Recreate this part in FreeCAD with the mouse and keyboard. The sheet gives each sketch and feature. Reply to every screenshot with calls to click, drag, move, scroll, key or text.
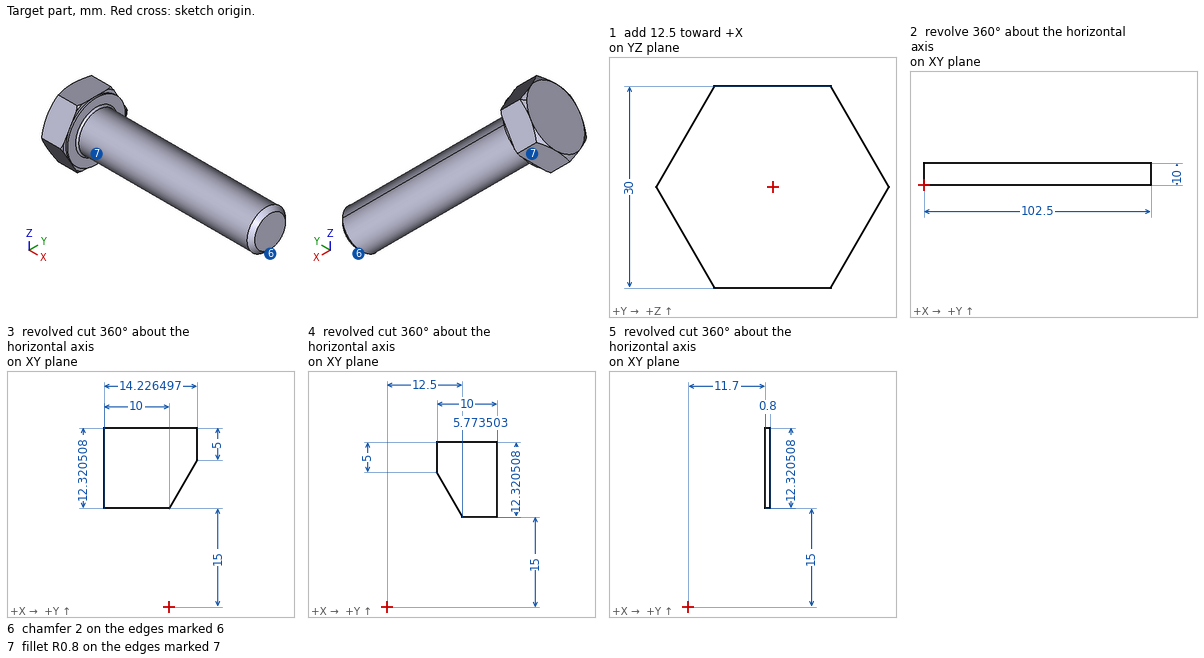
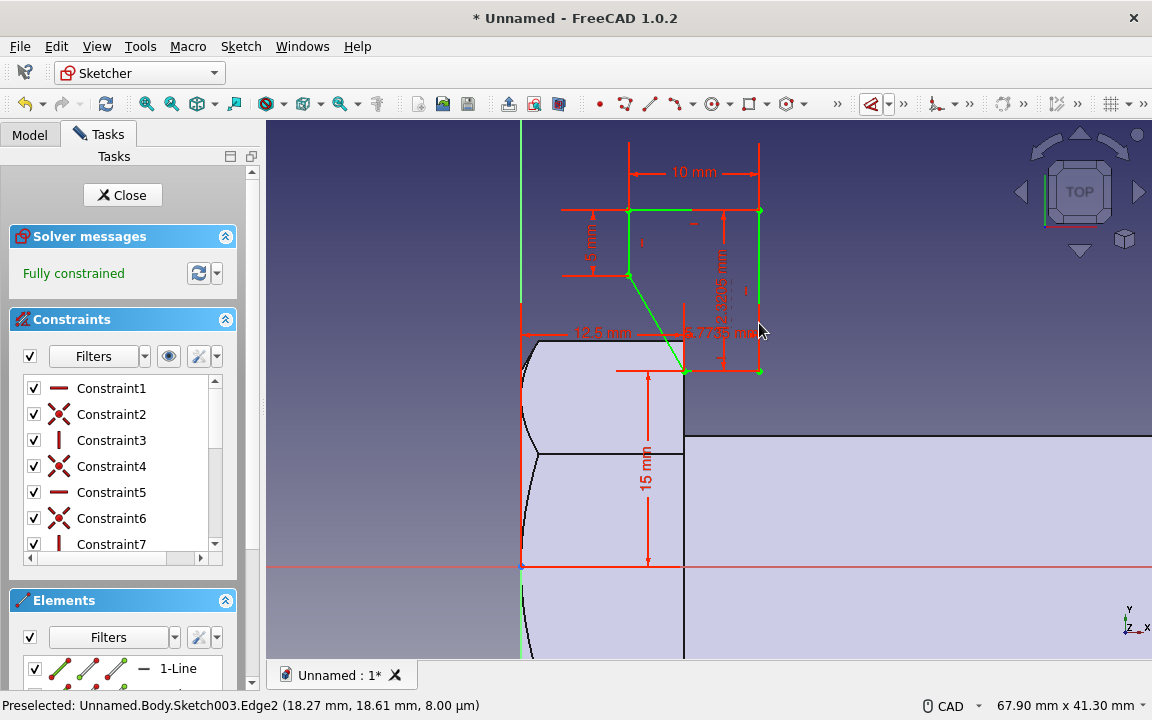
click(123, 195)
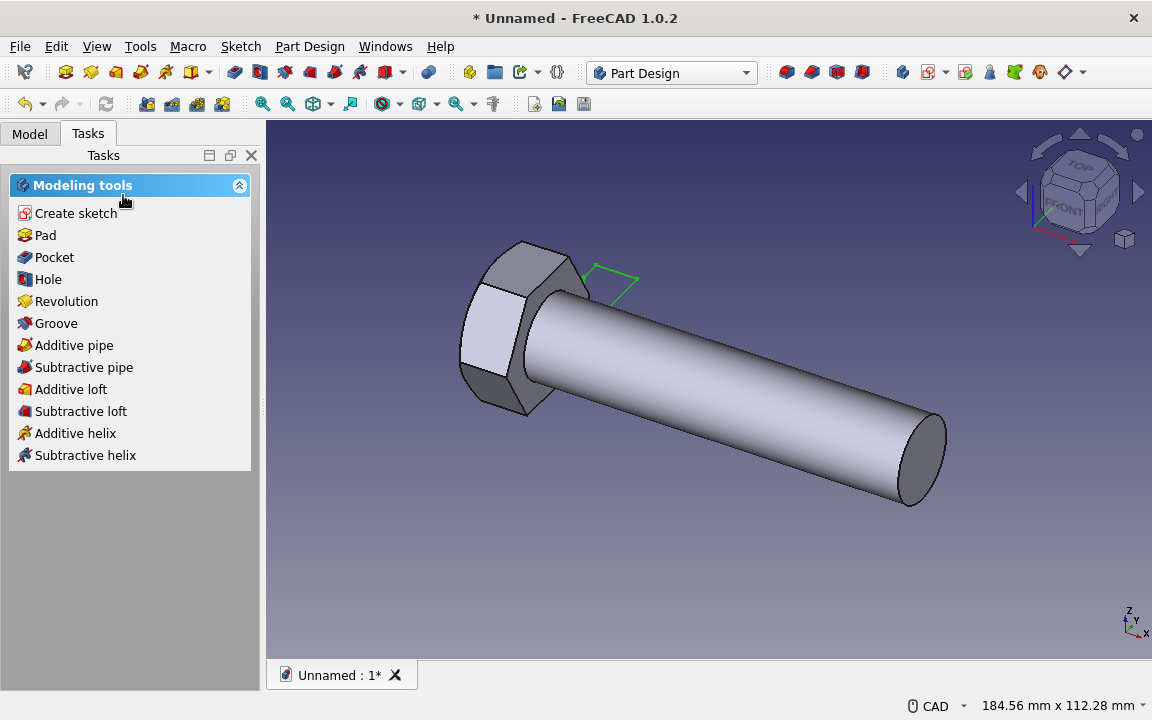
click(285, 72)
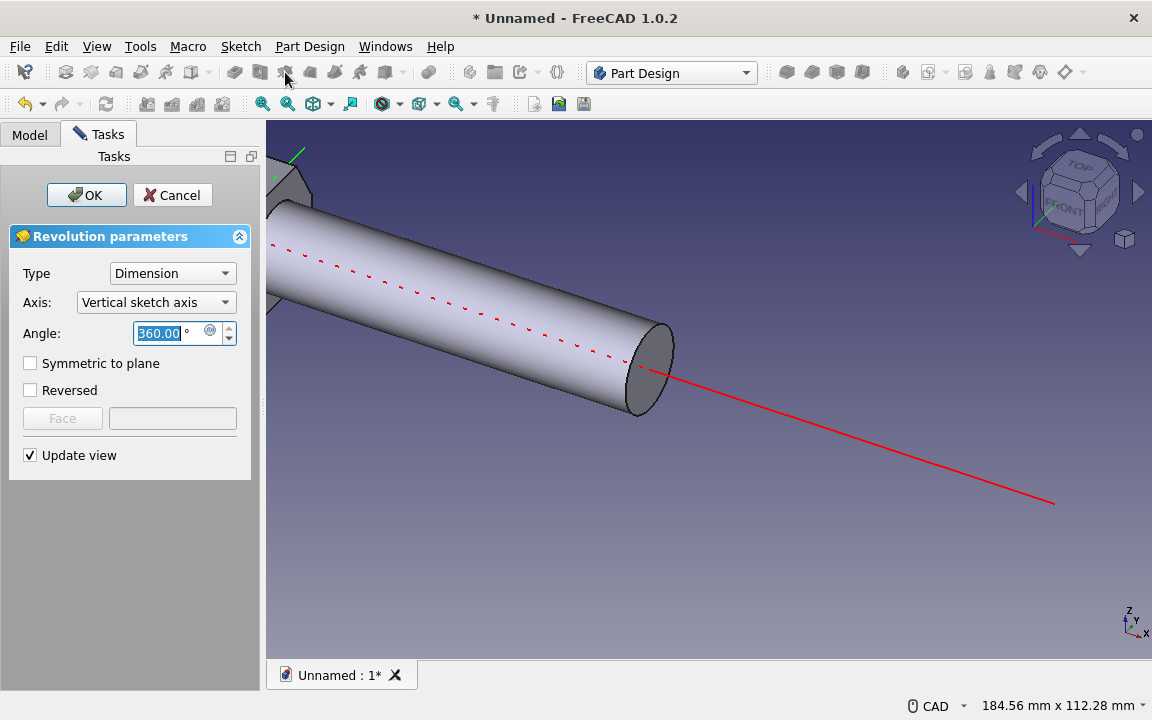
click(157, 302)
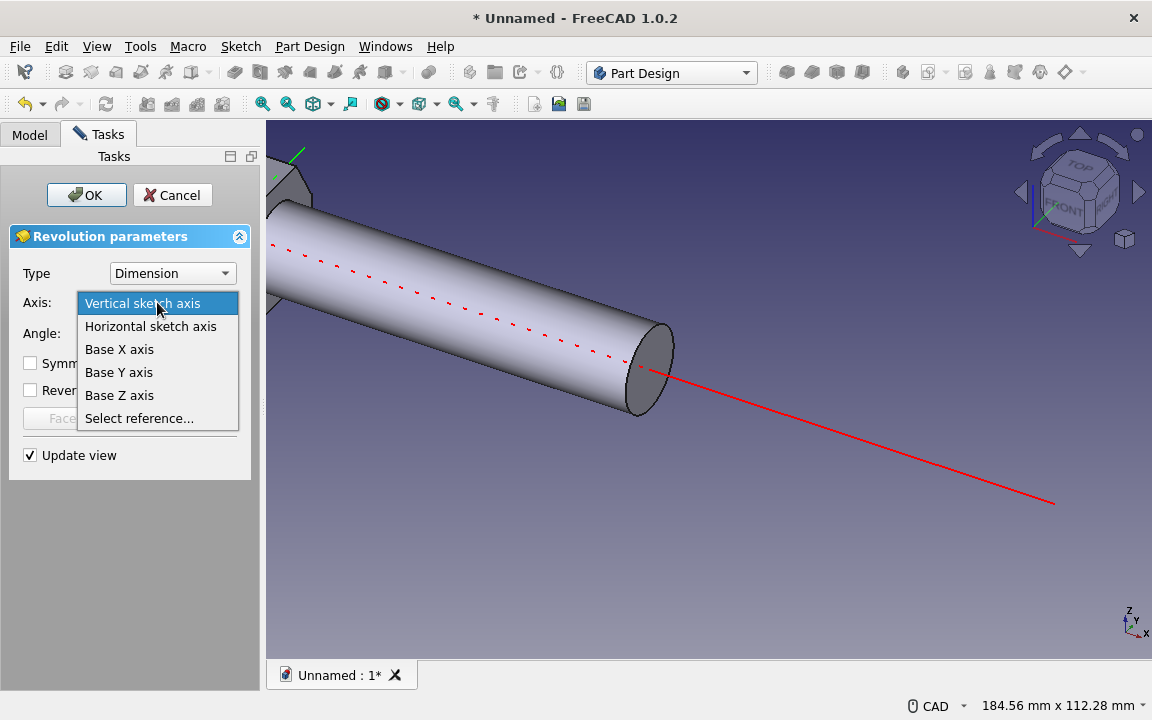
click(156, 326)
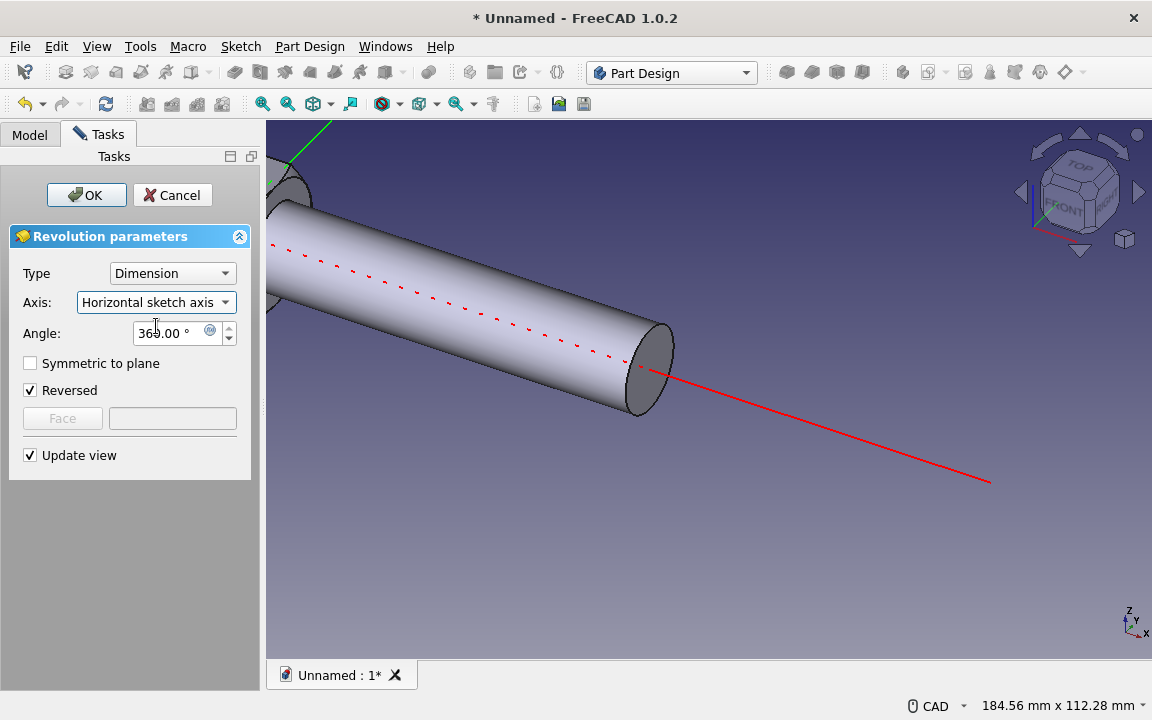
click(87, 195)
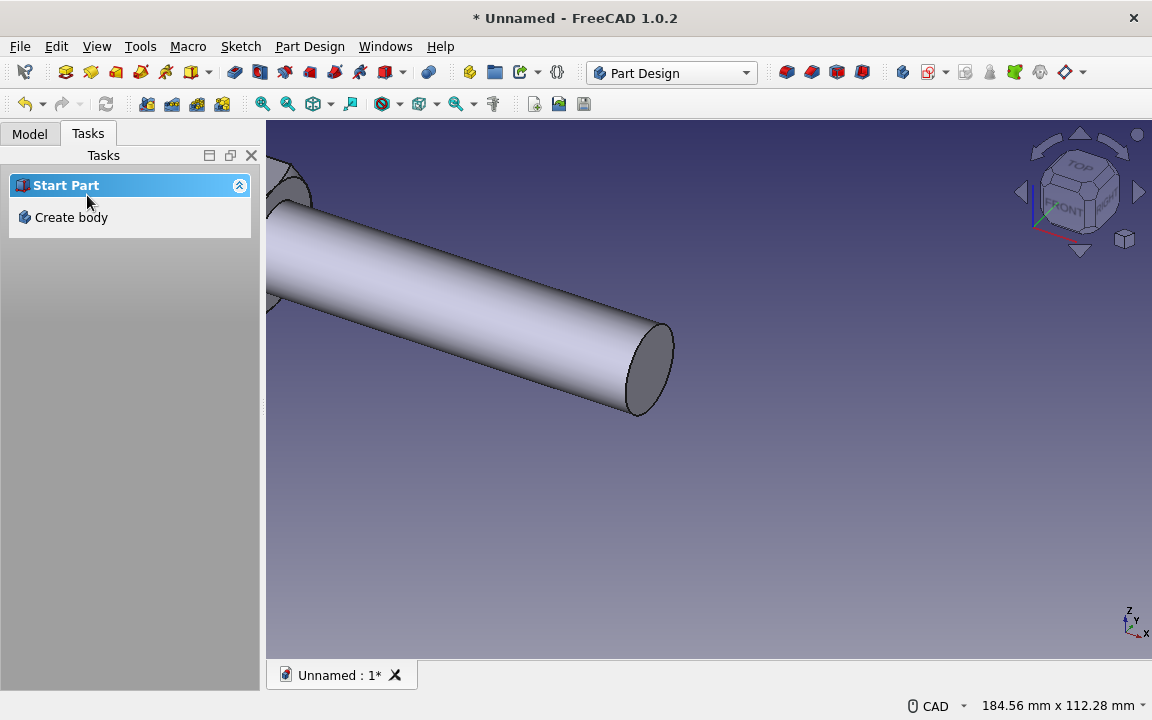
click(263, 104)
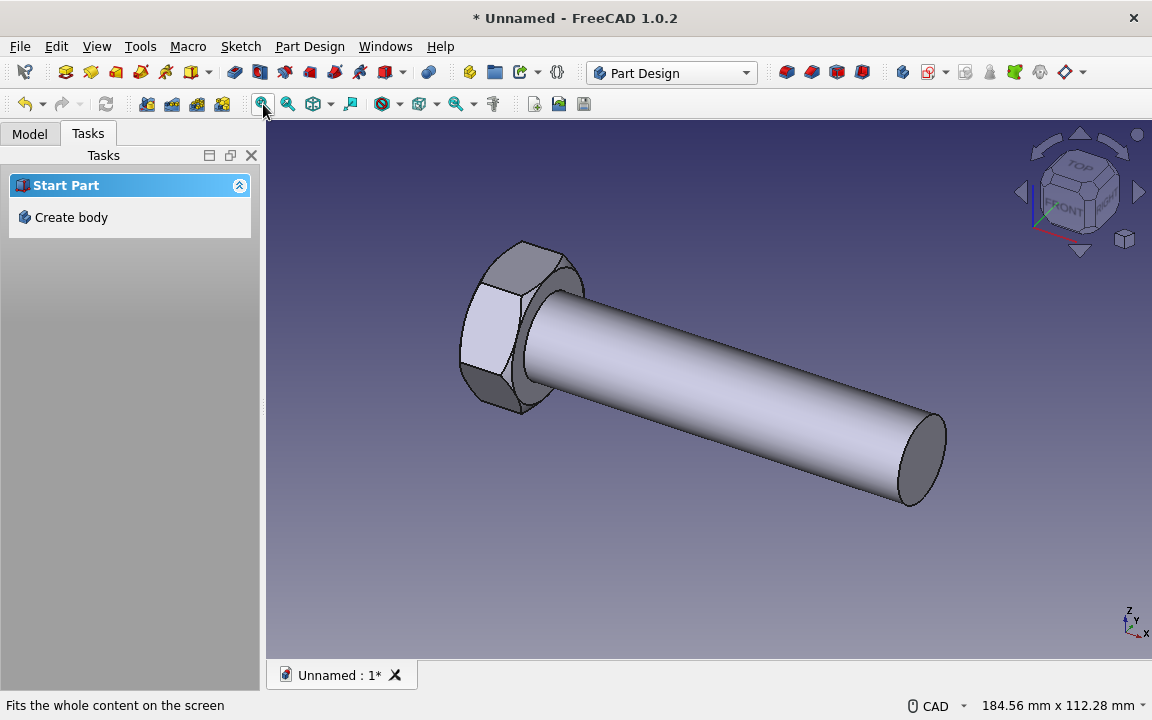
click(928, 72)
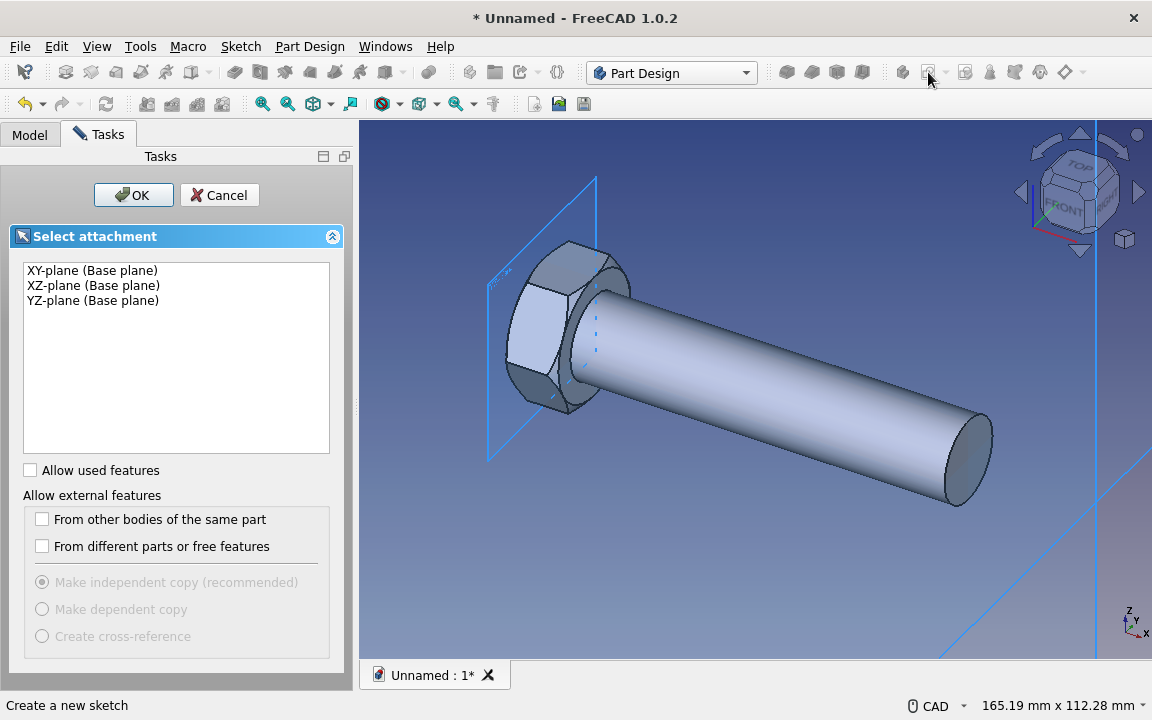
click(84, 270)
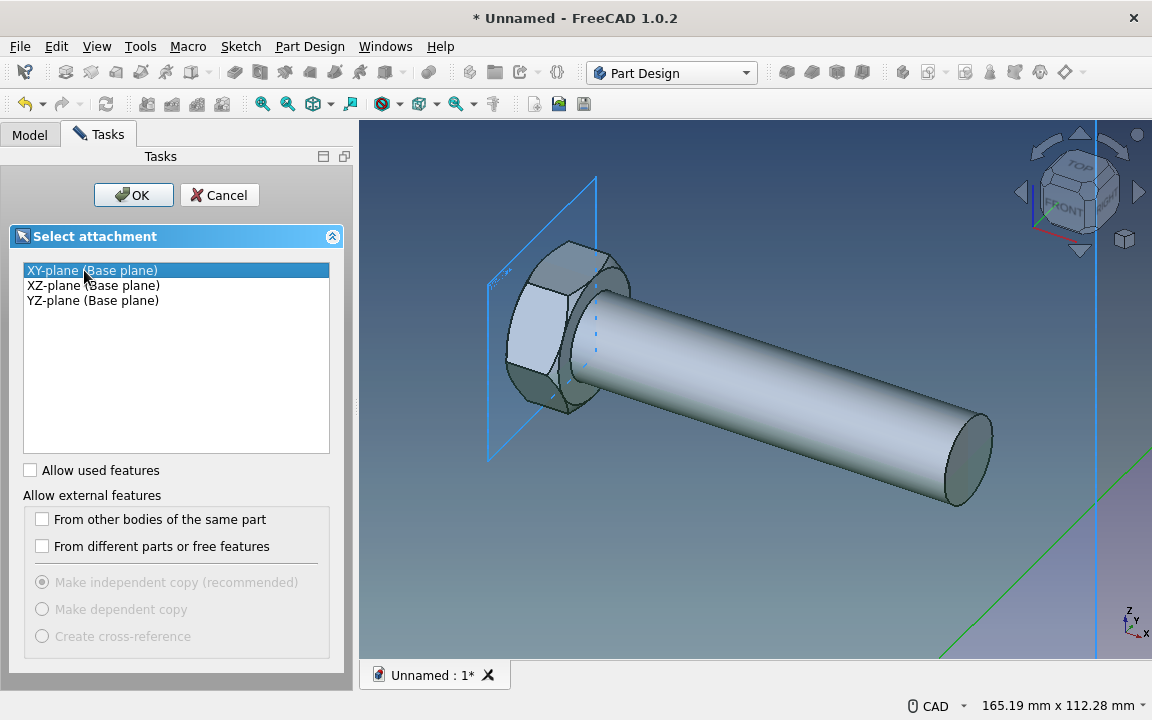
click(134, 195)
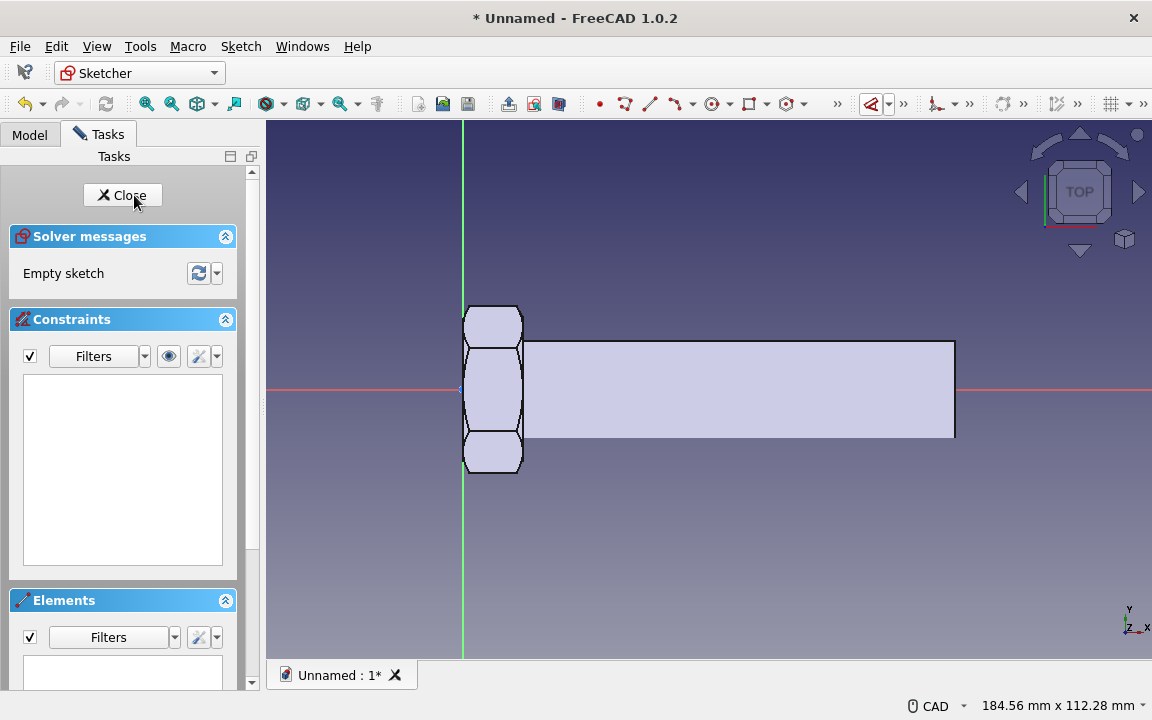
click(559, 104)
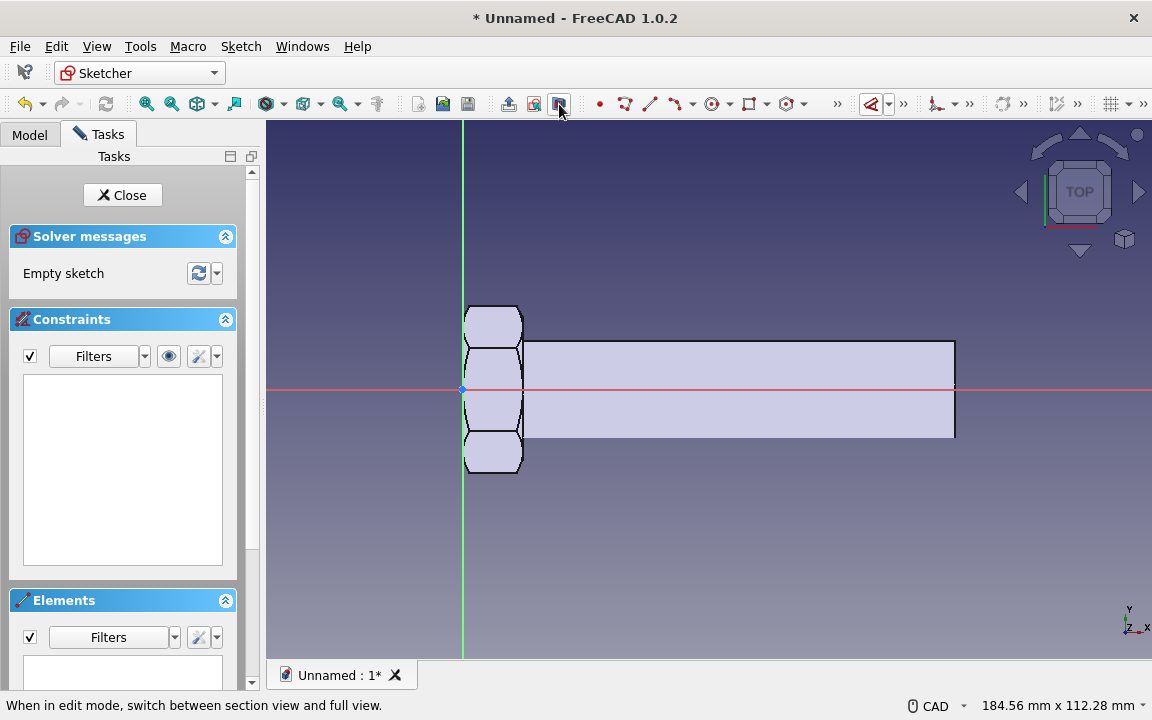
scroll(407, 286, up, 5)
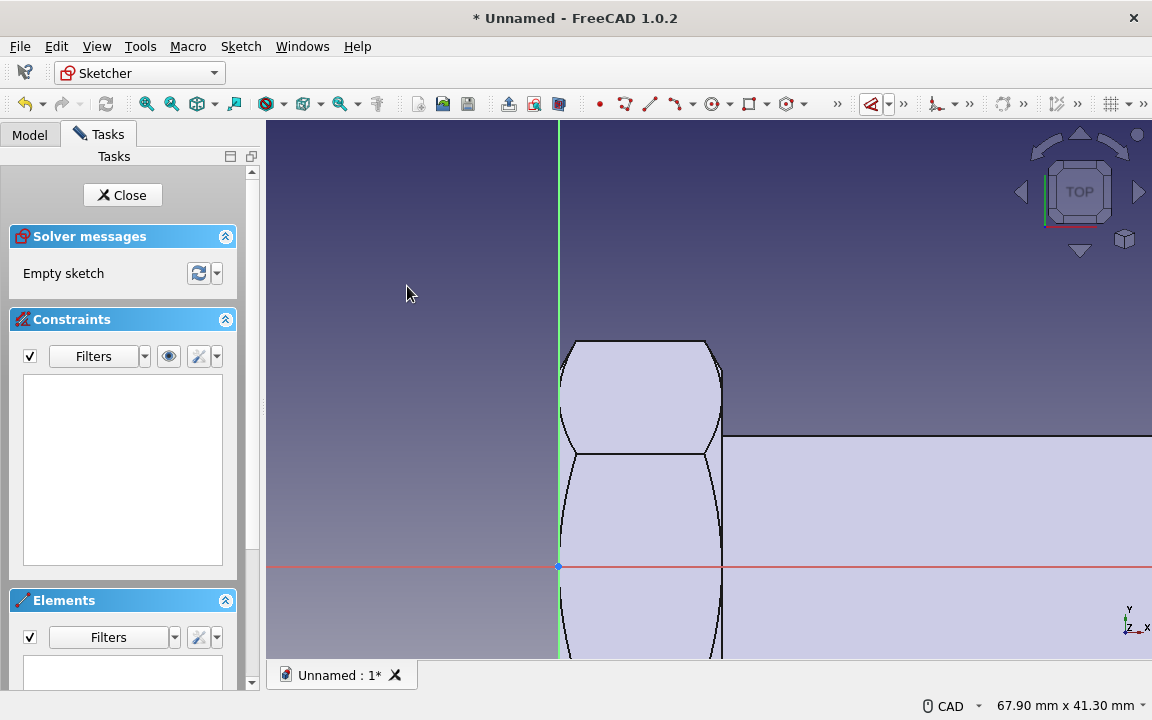
click(748, 104)